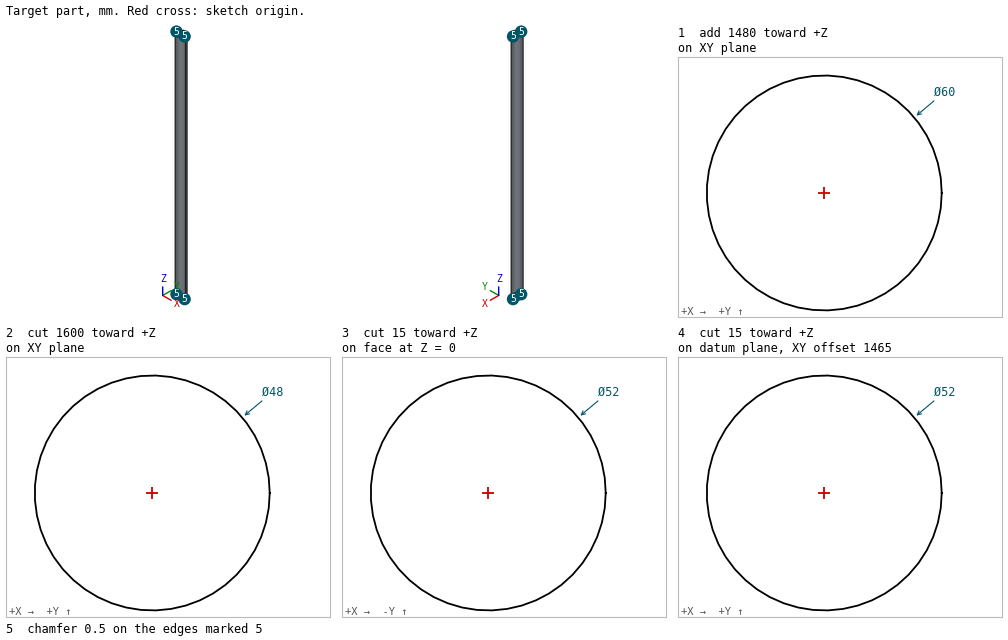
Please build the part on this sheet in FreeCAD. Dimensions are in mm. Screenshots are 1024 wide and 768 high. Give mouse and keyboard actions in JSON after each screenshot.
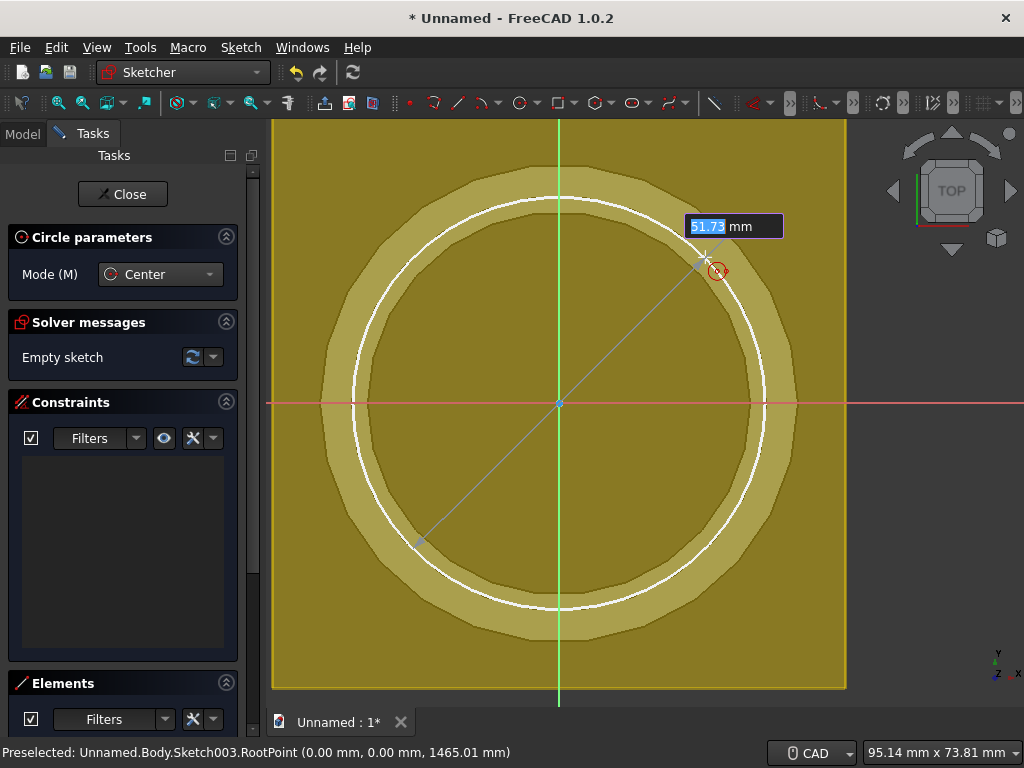
{"action": "type", "text": "52"}
{"action": "key", "text": "Return"}
{"action": "key", "text": "Escape"}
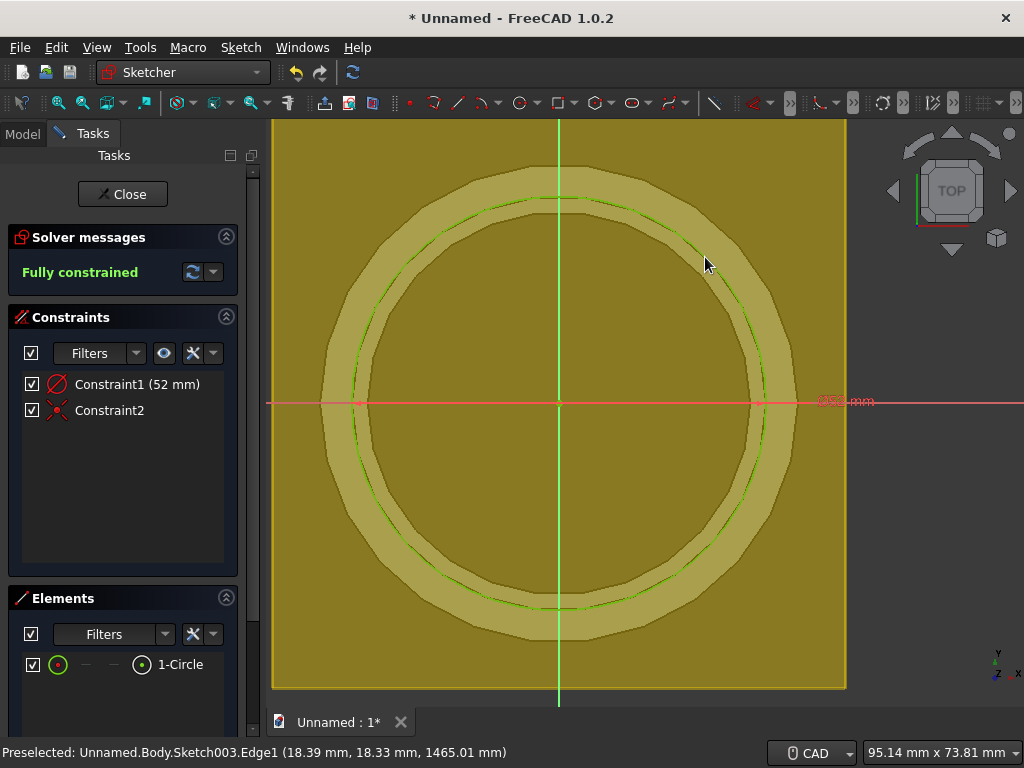
{"action": "left_click", "coordinate": [123, 194]}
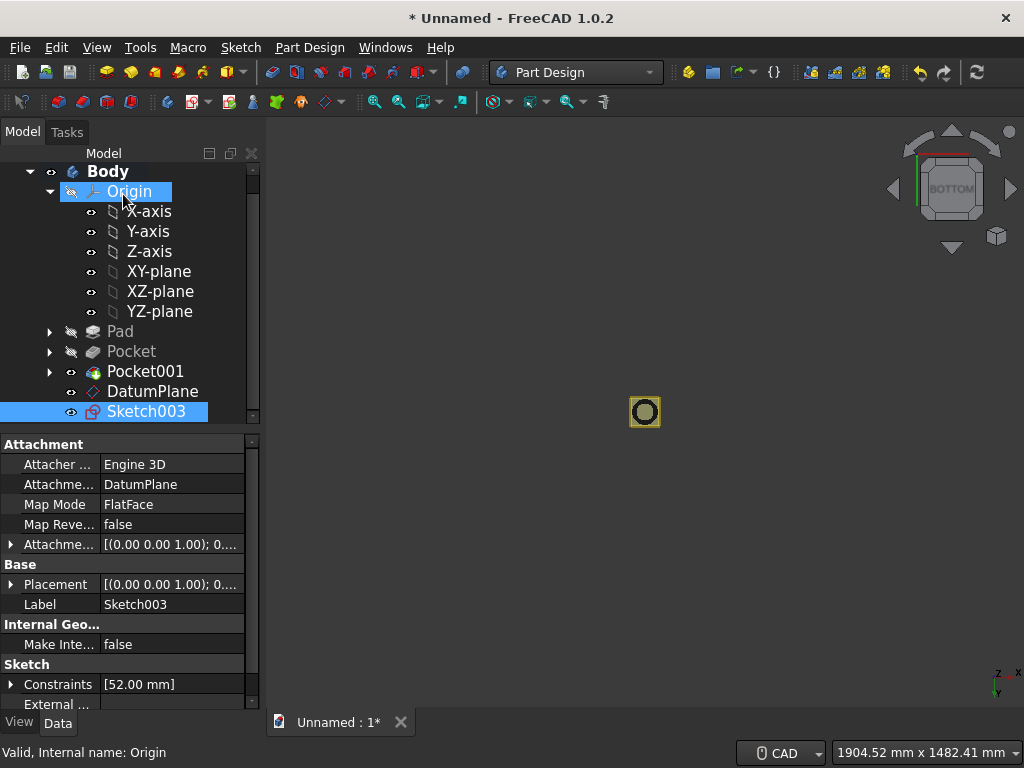
{"action": "left_click", "coordinate": [274, 72]}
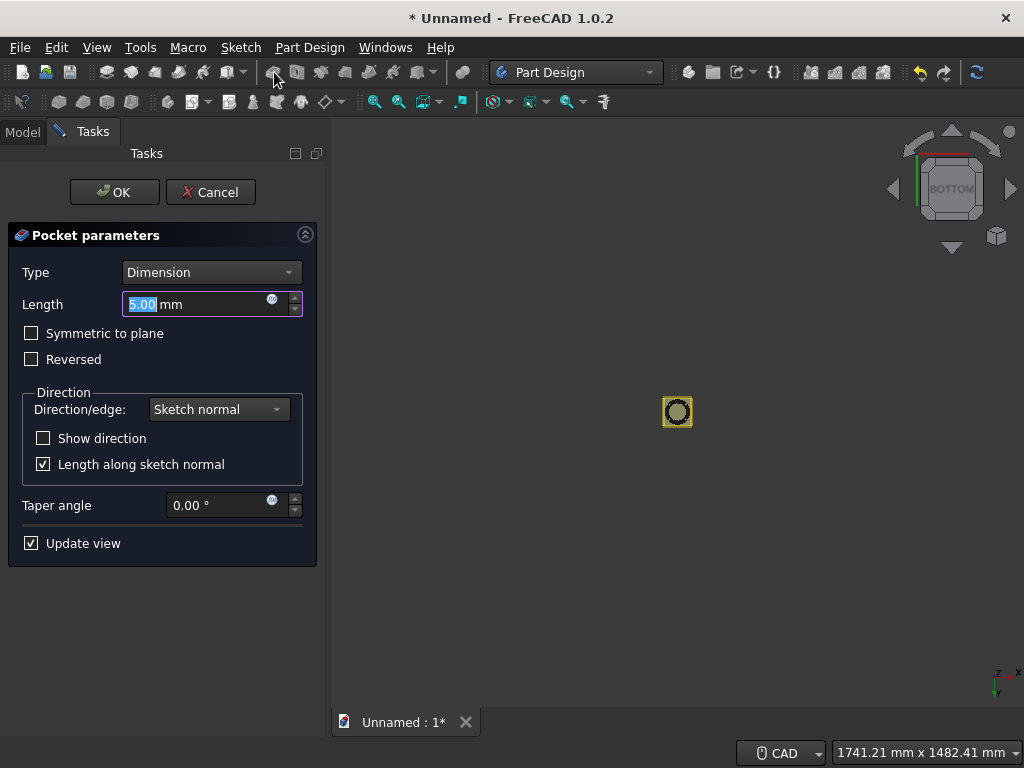
{"action": "type", "text": "15"}
{"action": "key", "text": "Tab"}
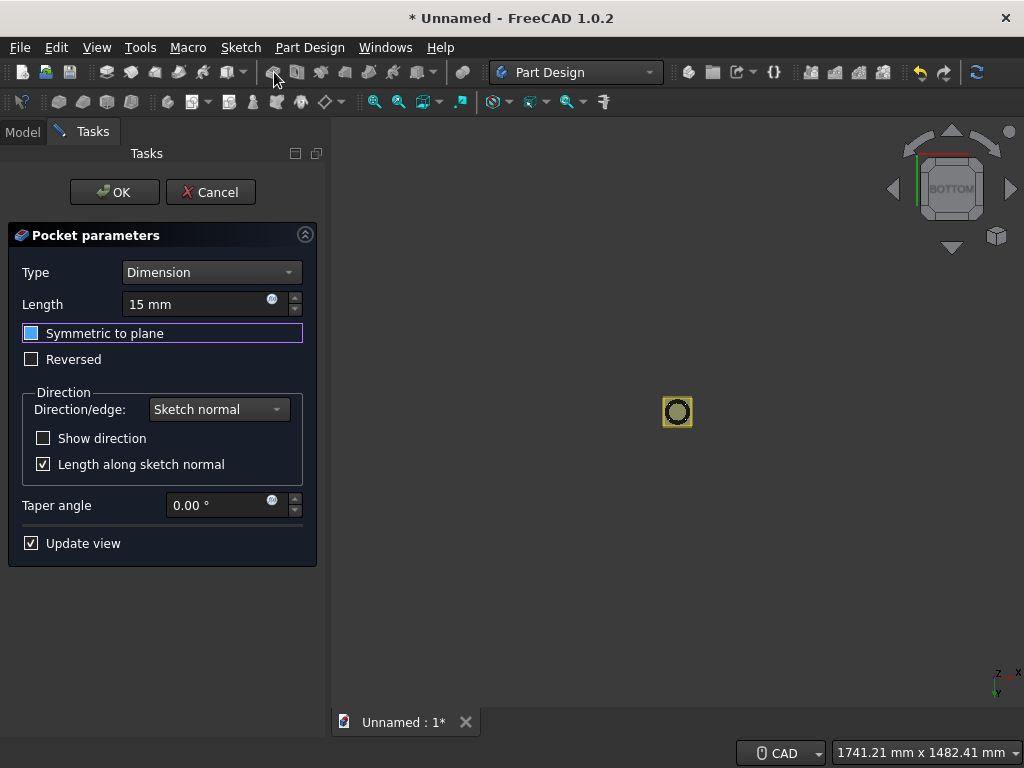
{"action": "left_click", "coordinate": [30, 359]}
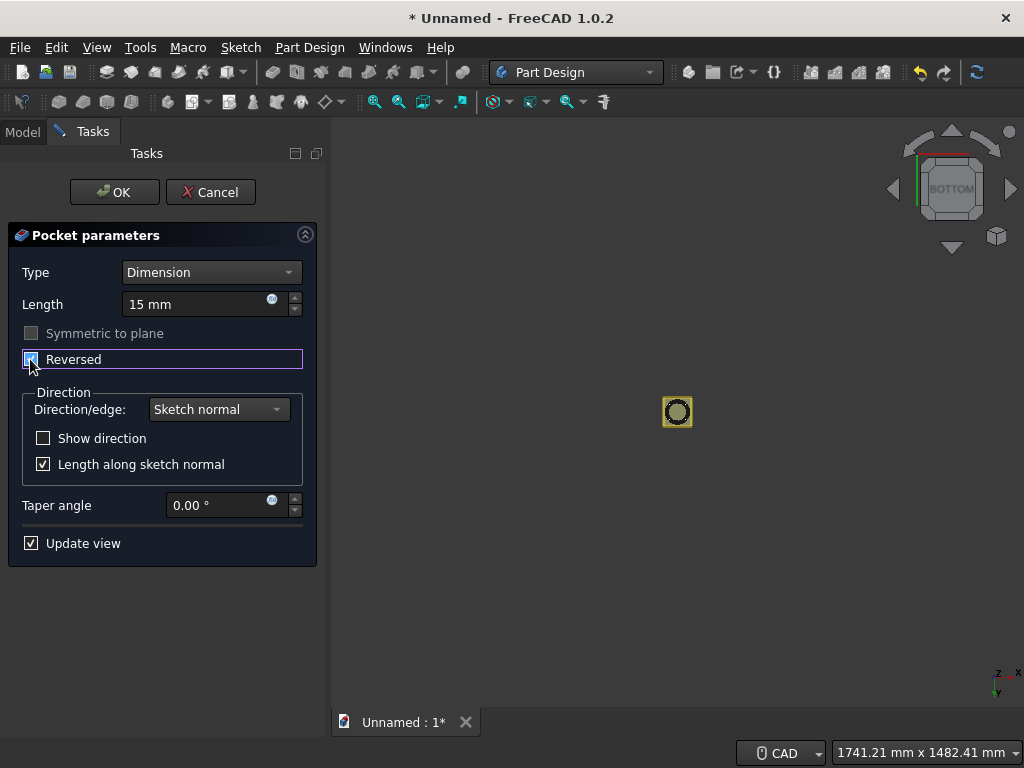
{"action": "left_click", "coordinate": [115, 192]}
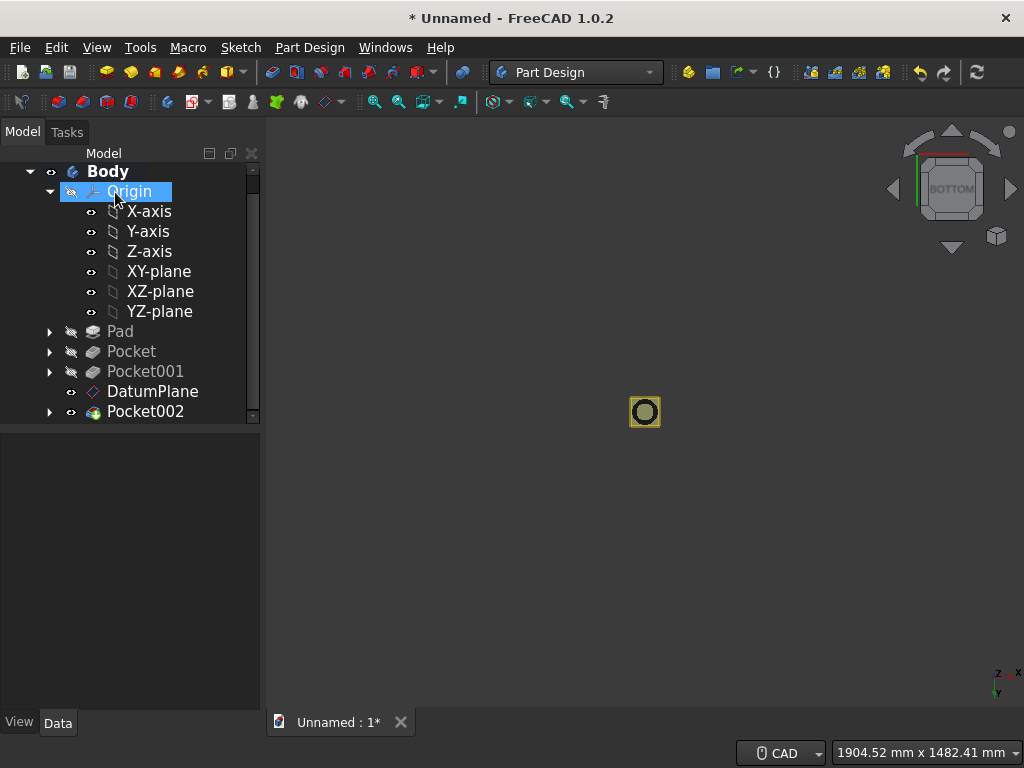
{"action": "left_click", "coordinate": [116, 392]}
{"action": "key", "text": "space"}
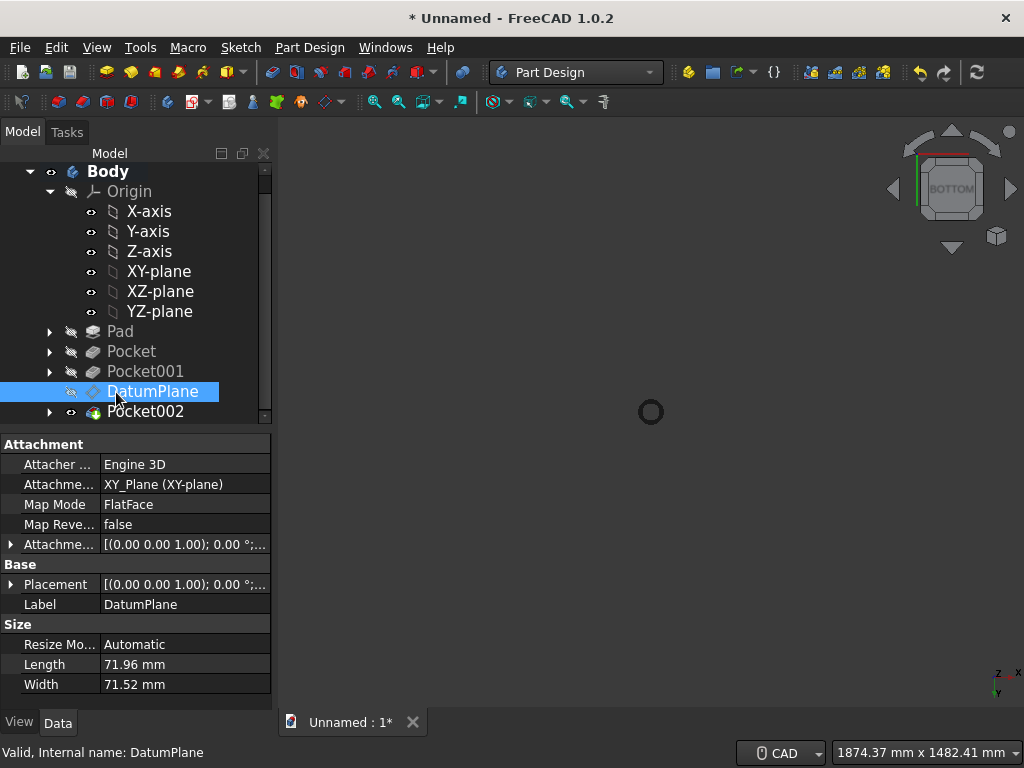
{"action": "left_click", "coordinate": [376, 102]}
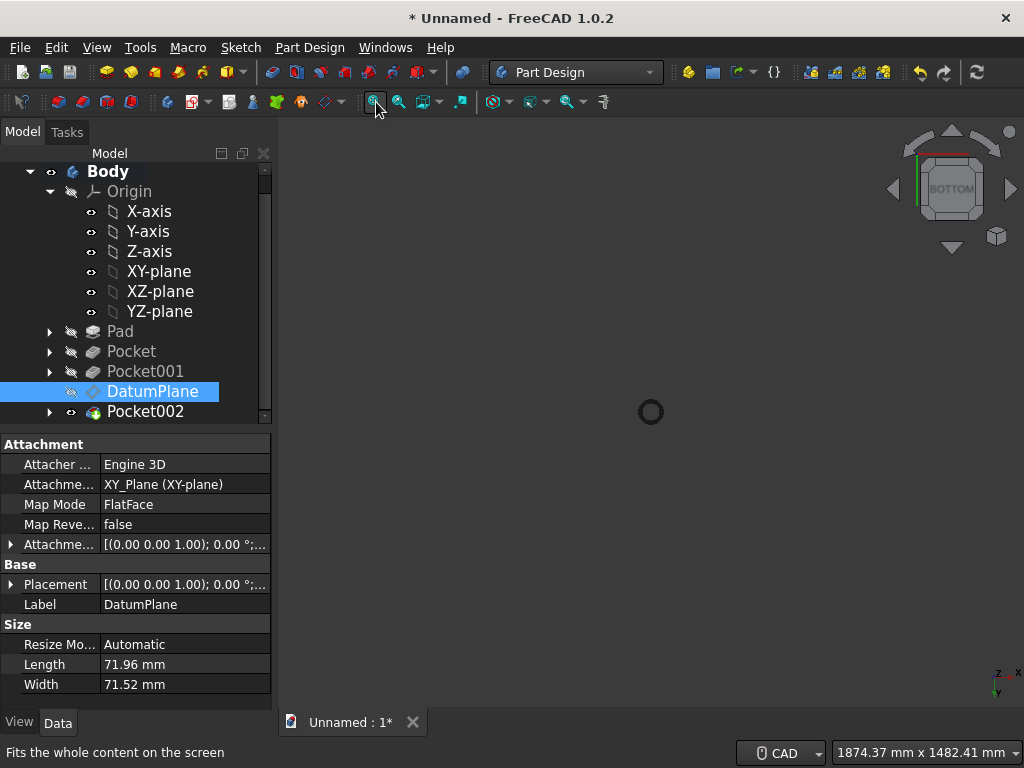
{"action": "left_click", "coordinate": [643, 405]}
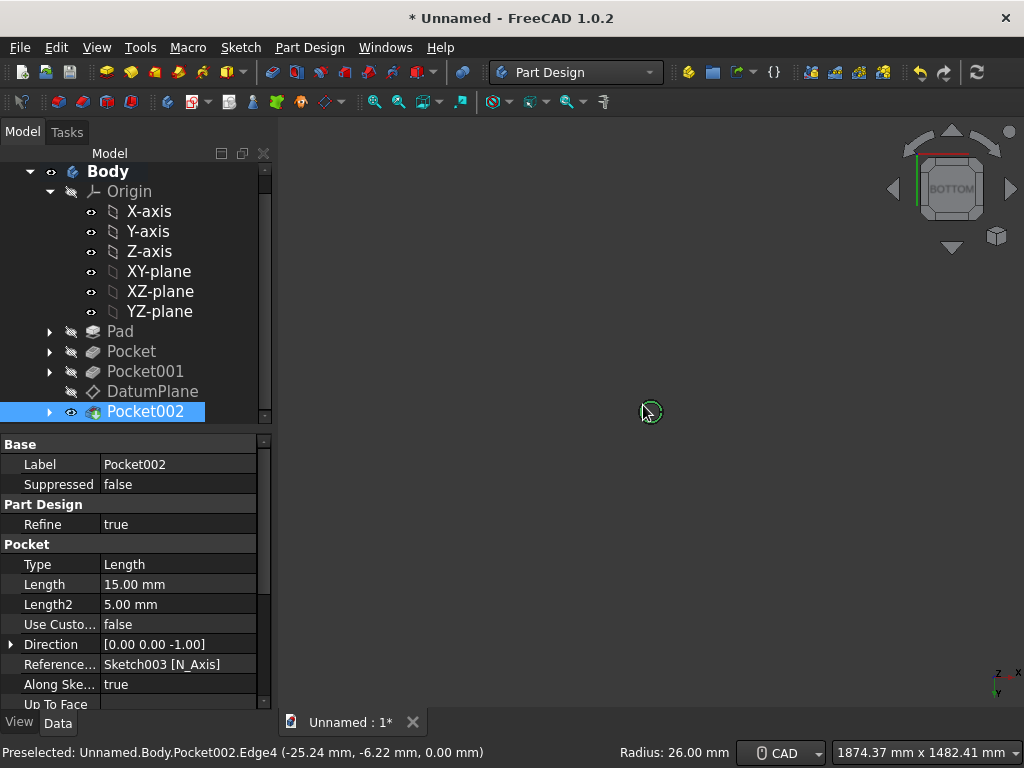
{"action": "left_click", "coordinate": [639, 411], "text": "ctrl"}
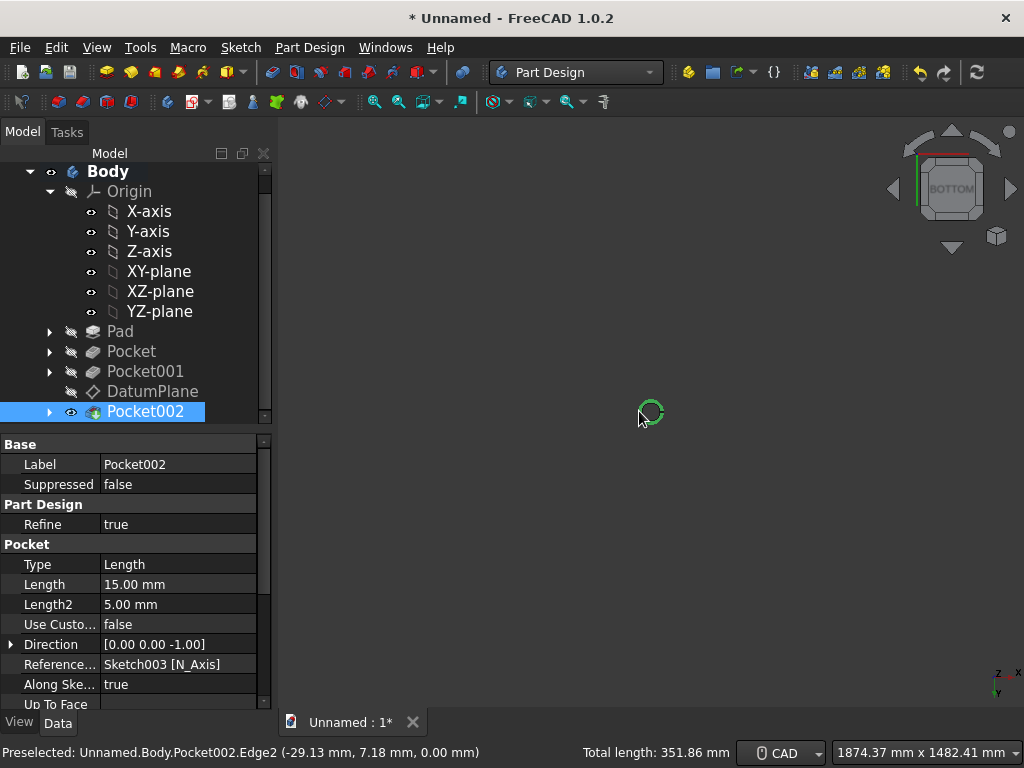
{"action": "key", "text": "0"}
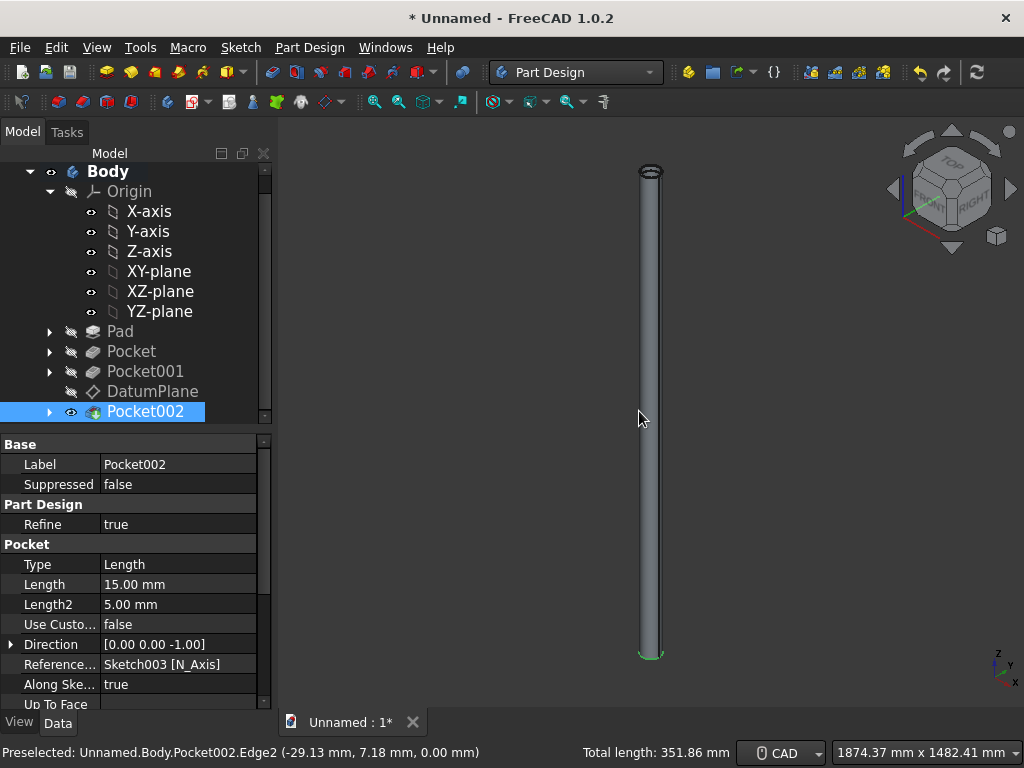
{"action": "left_click", "coordinate": [644, 166], "text": "ctrl"}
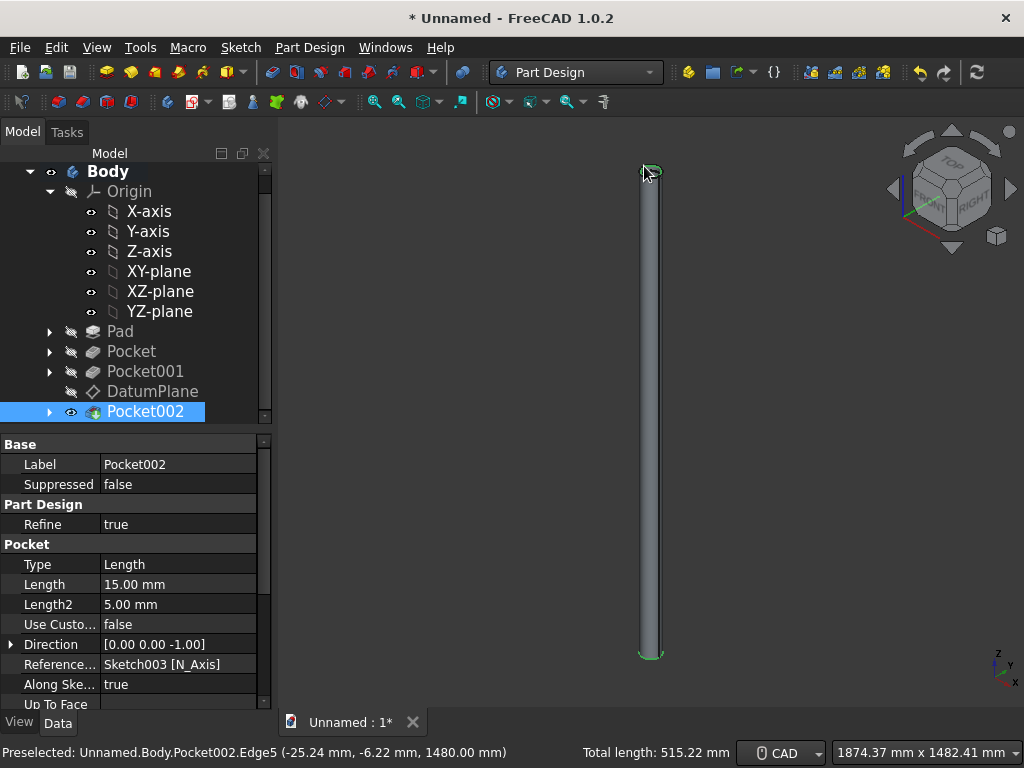
{"action": "left_click", "coordinate": [640, 174], "text": "ctrl"}